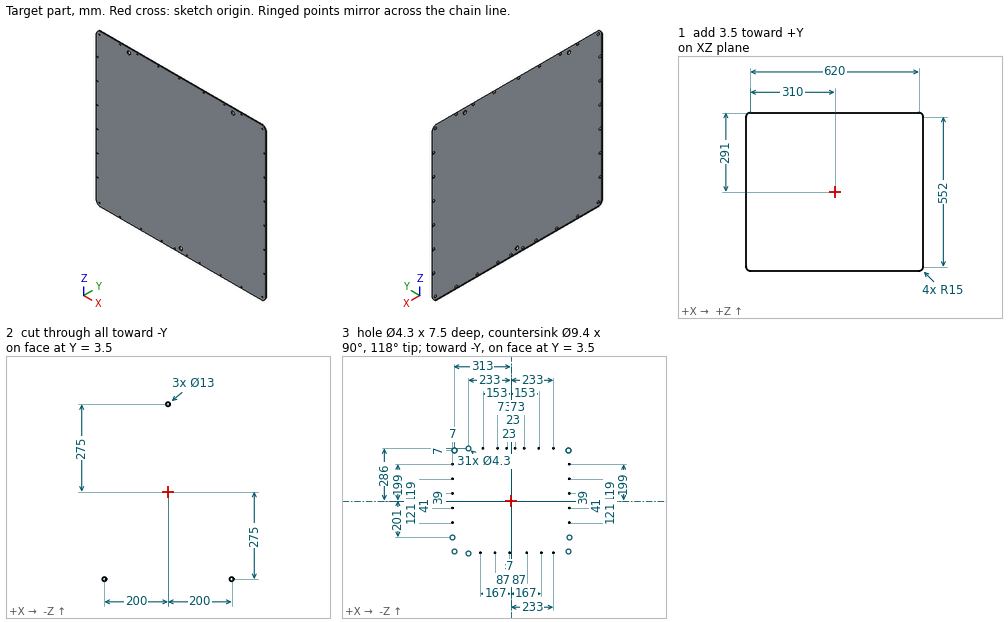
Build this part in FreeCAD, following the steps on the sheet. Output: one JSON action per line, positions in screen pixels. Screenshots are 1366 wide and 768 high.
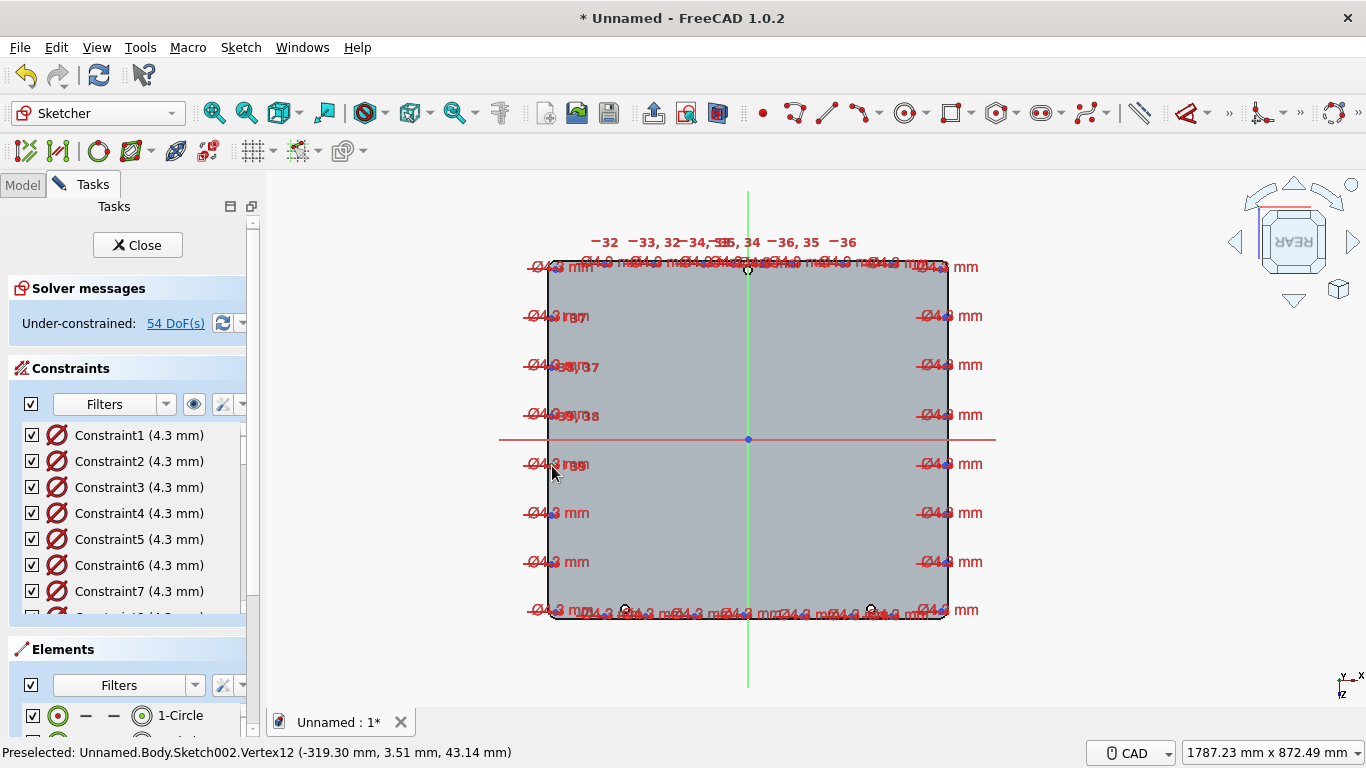
{"action": "left_click", "coordinate": [552, 515]}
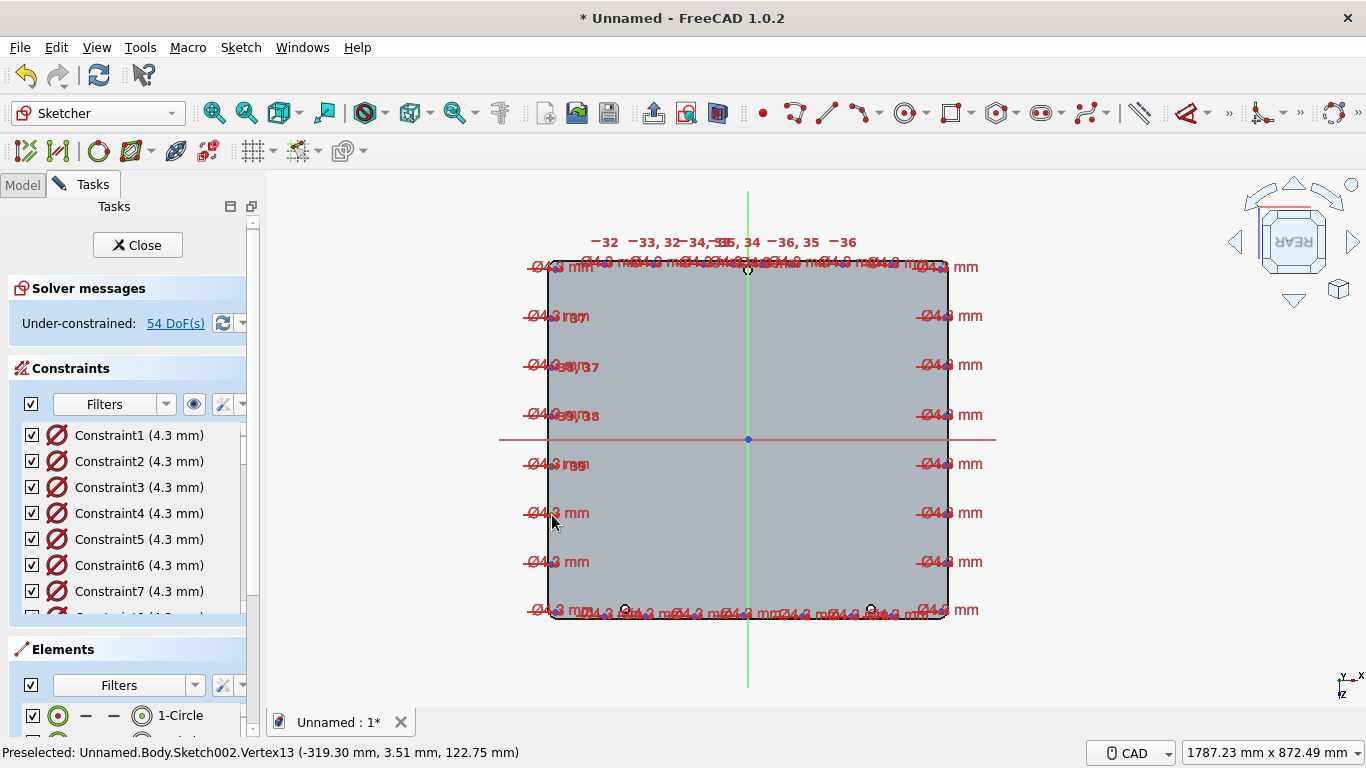
{"action": "key", "text": "v"}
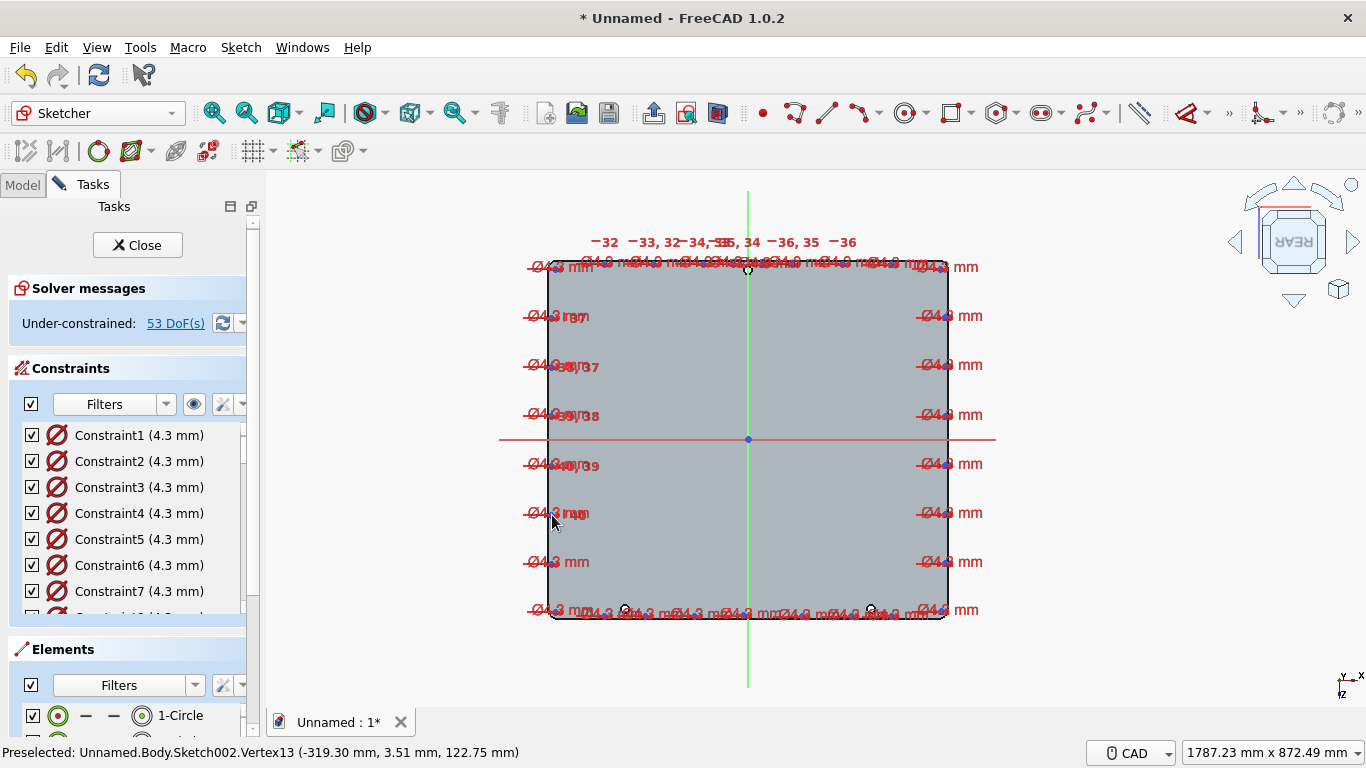
{"action": "left_click", "coordinate": [552, 515]}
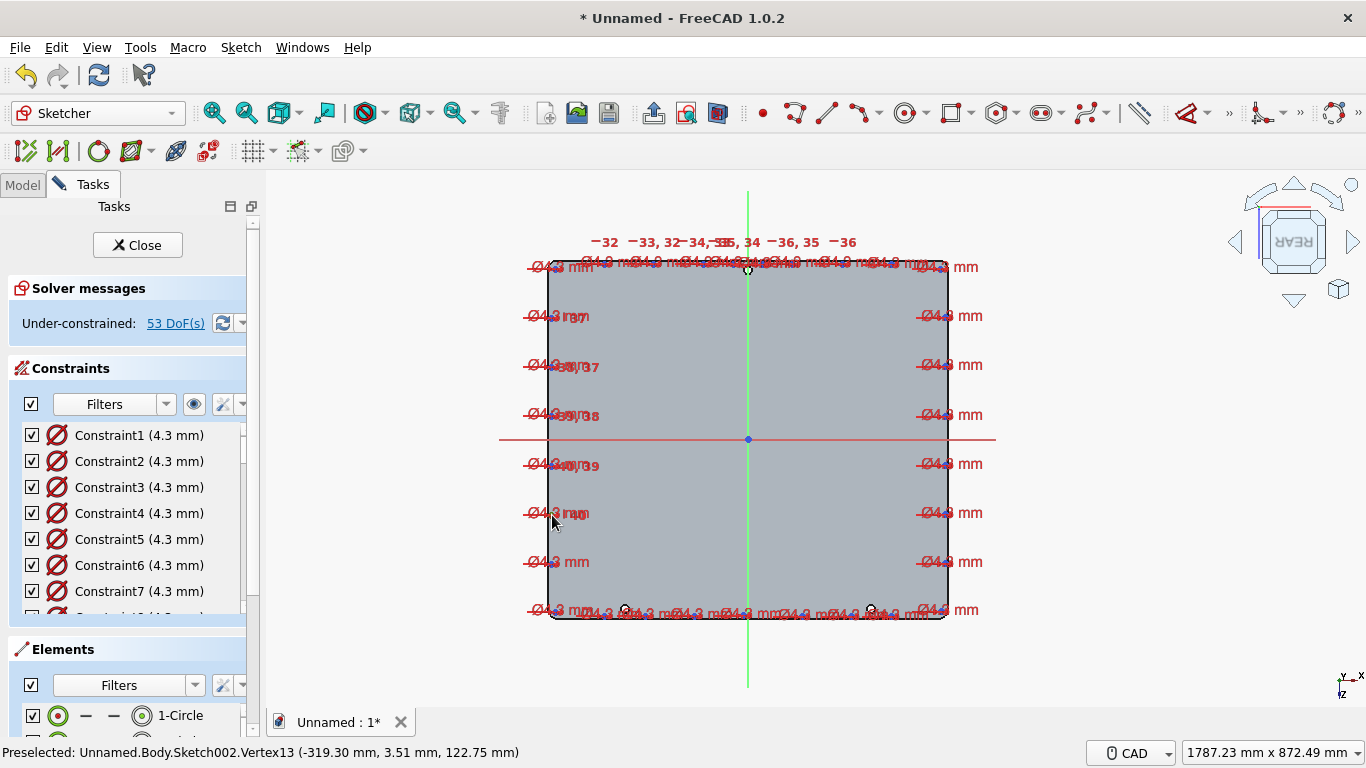
{"action": "left_click", "coordinate": [552, 564]}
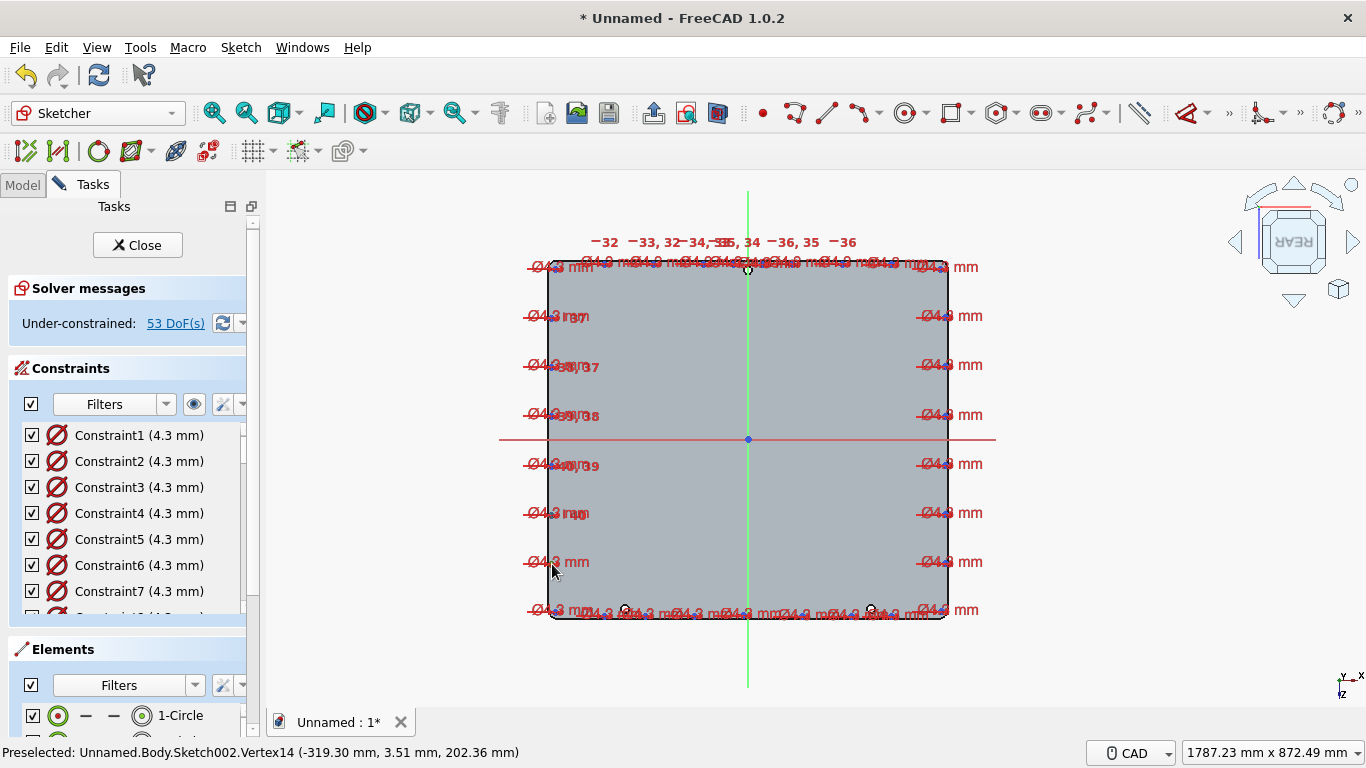
{"action": "key", "text": "v"}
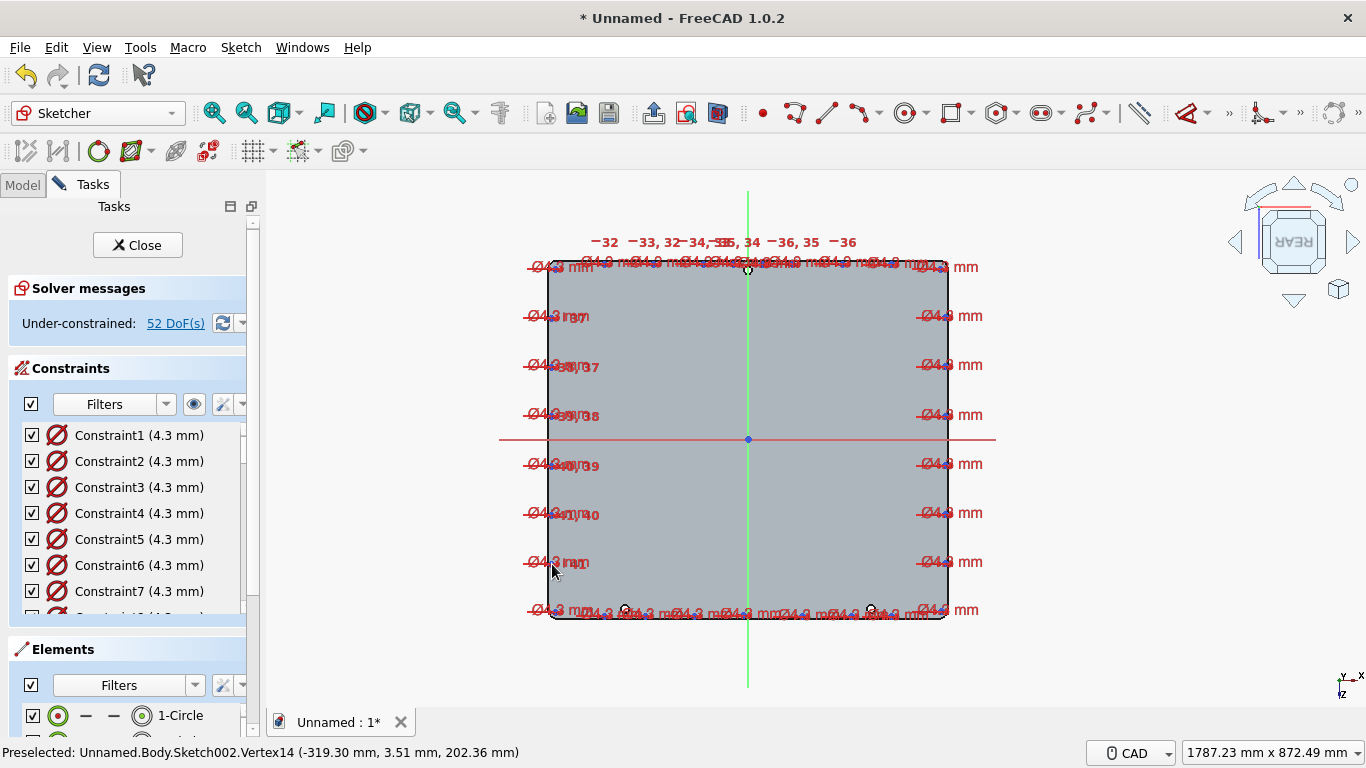
{"action": "left_click", "coordinate": [605, 616]}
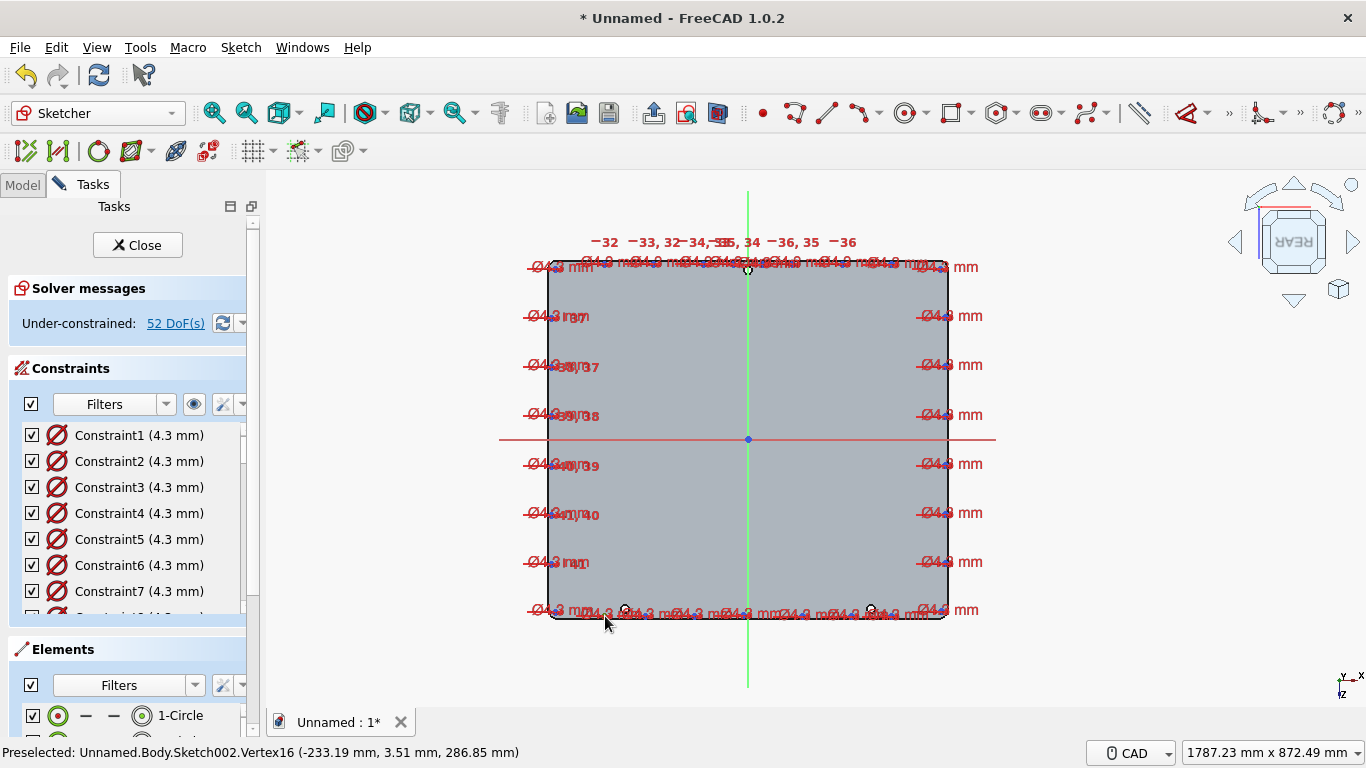
{"action": "left_click", "coordinate": [646, 616]}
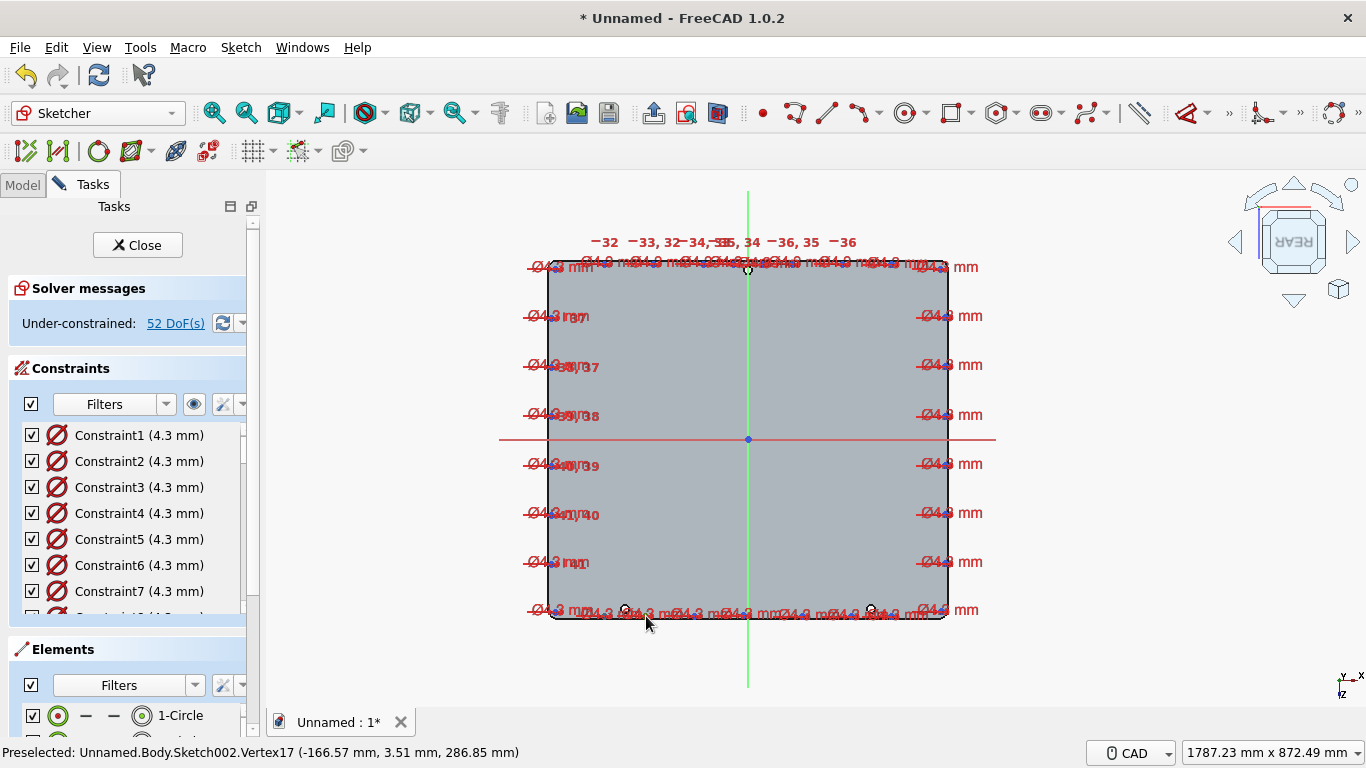
{"action": "key", "text": "h"}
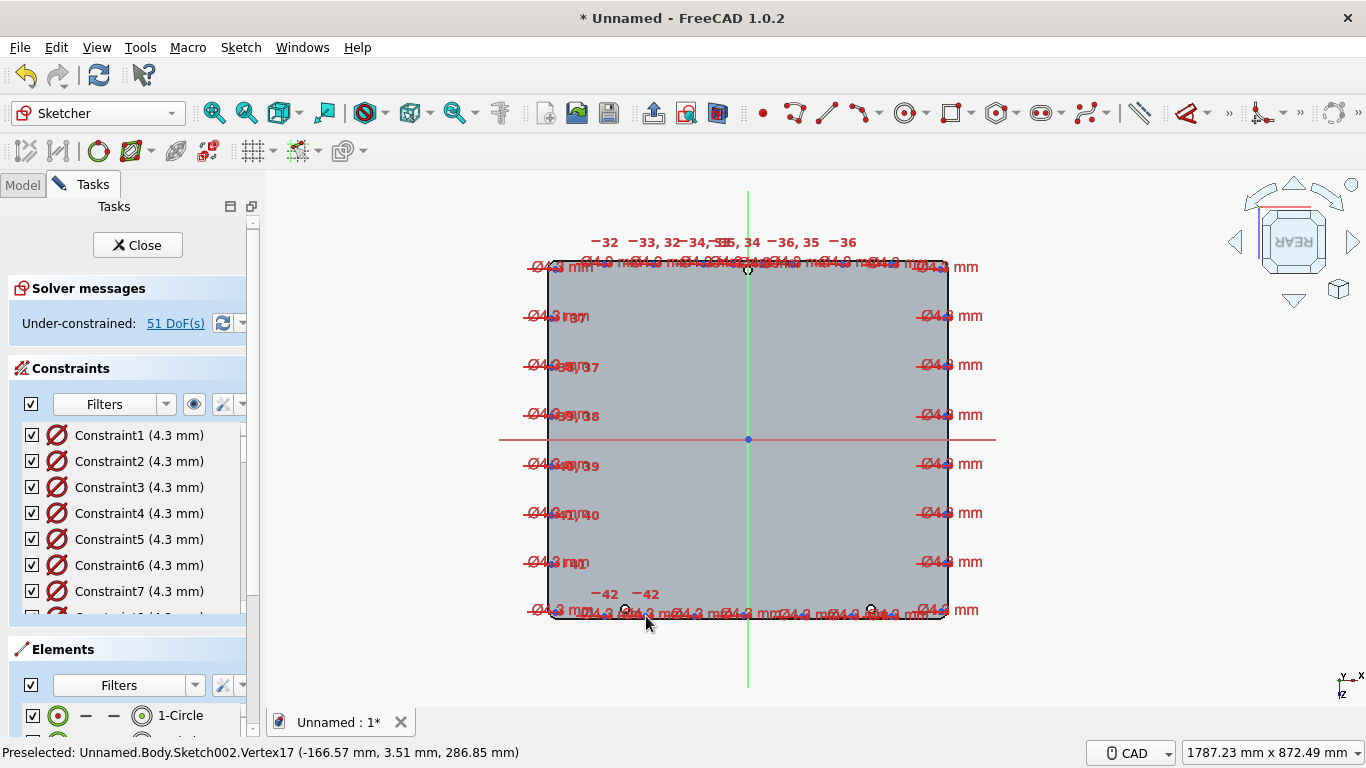
{"action": "left_click", "coordinate": [646, 616]}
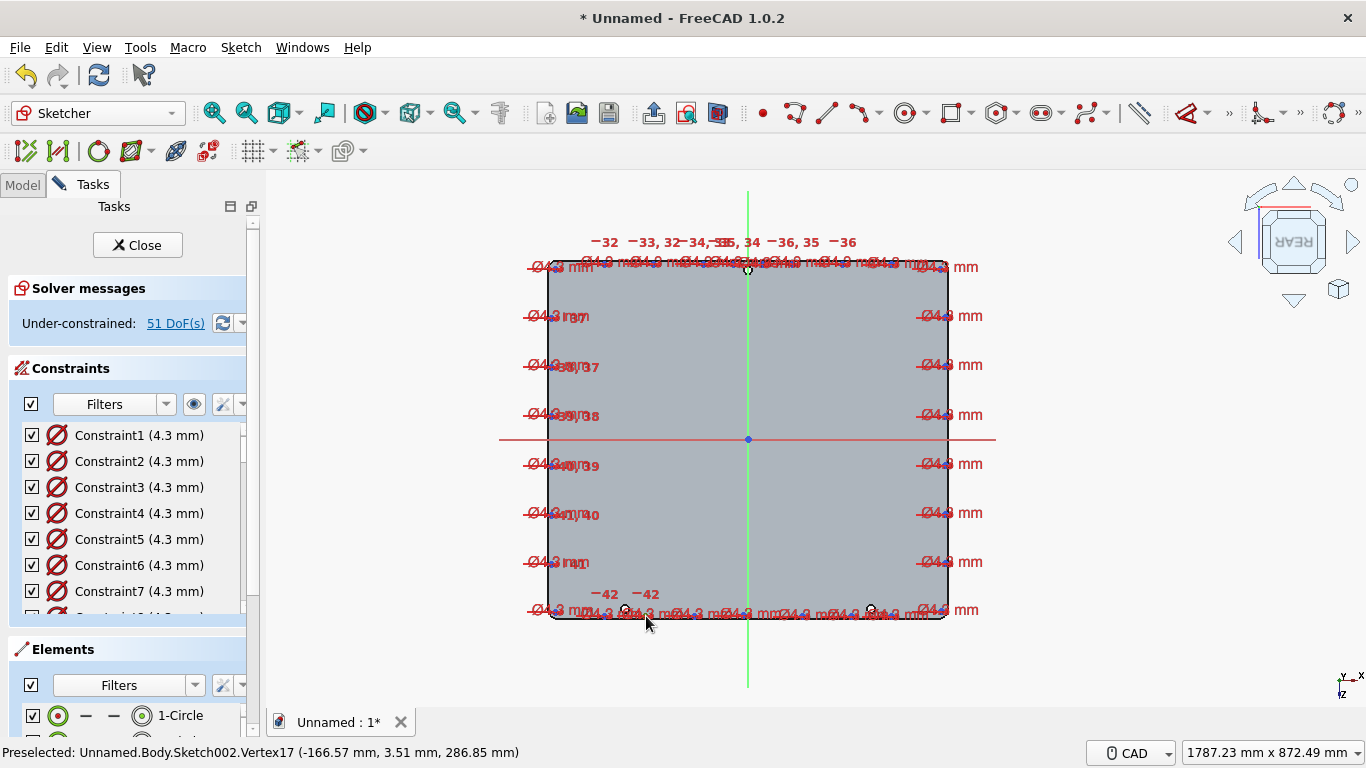
{"action": "left_click", "coordinate": [695, 616]}